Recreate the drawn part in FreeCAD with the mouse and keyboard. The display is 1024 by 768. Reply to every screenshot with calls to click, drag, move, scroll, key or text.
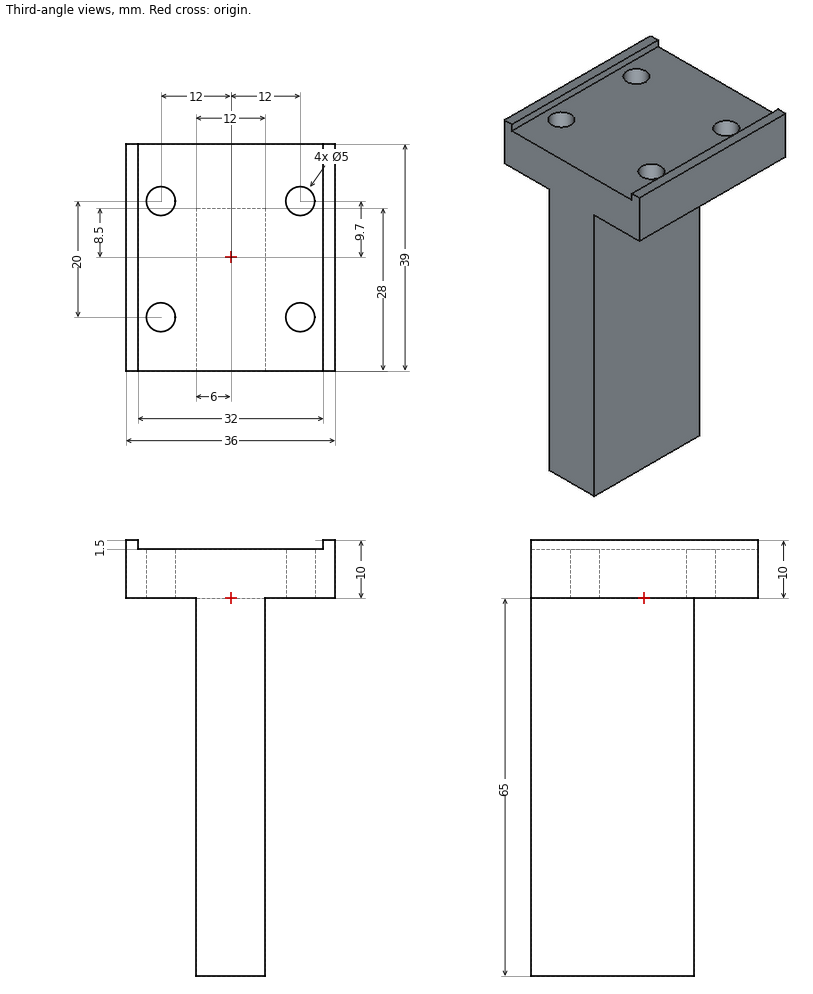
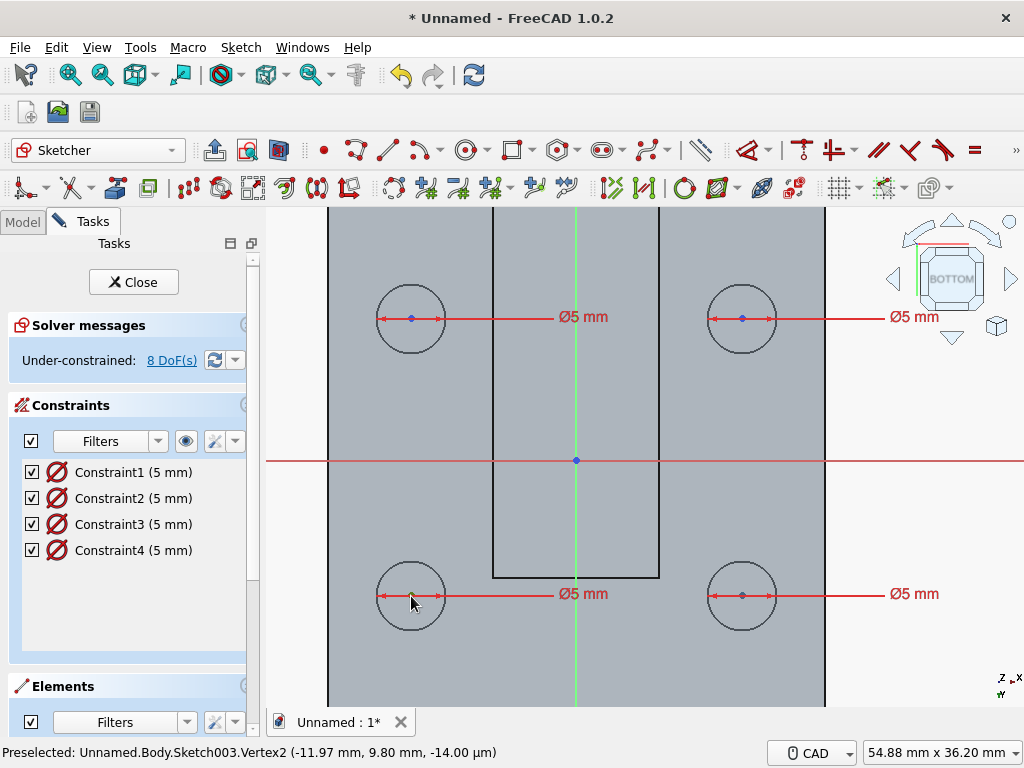
key(h)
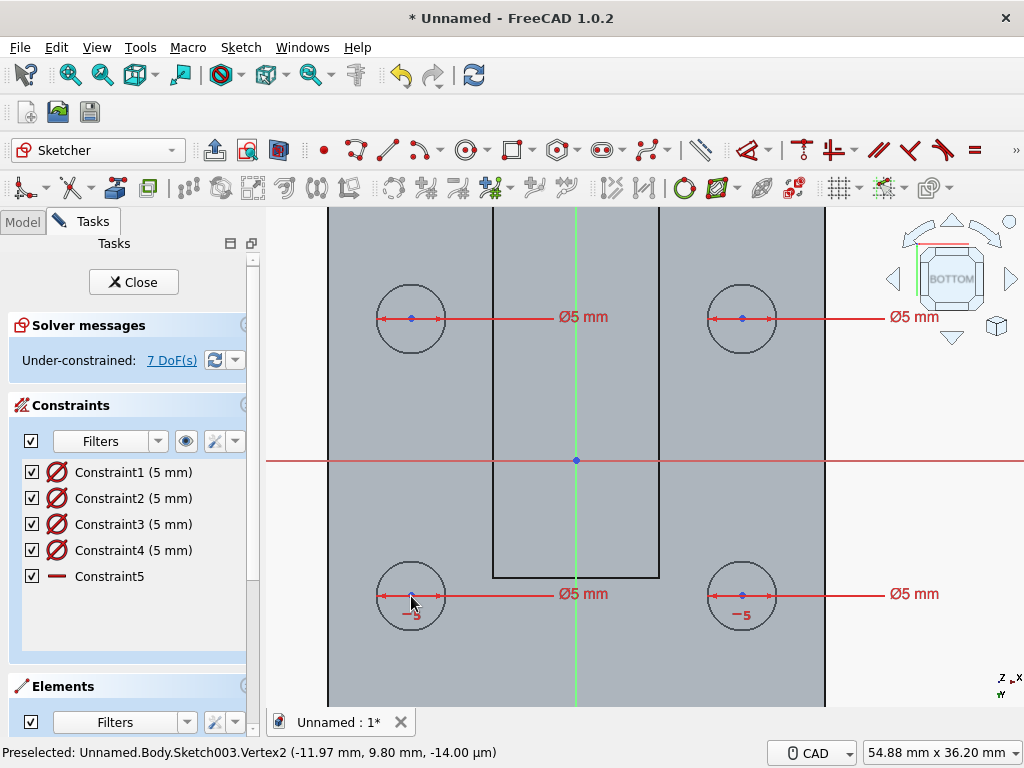
click(411, 596)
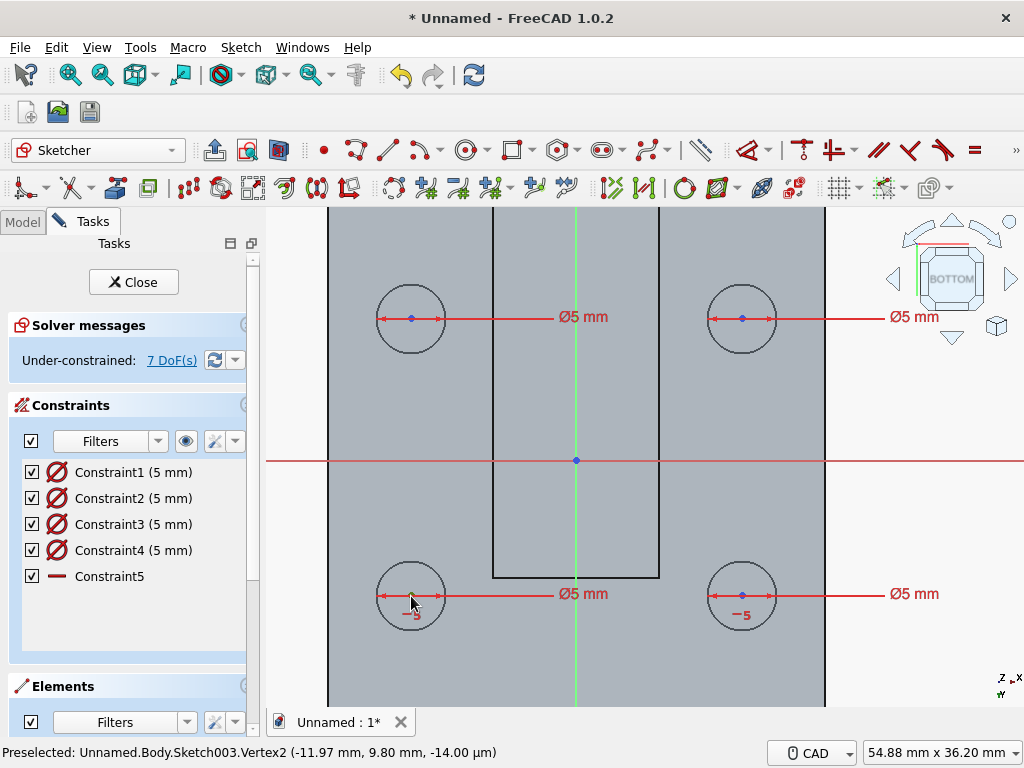
click(411, 319)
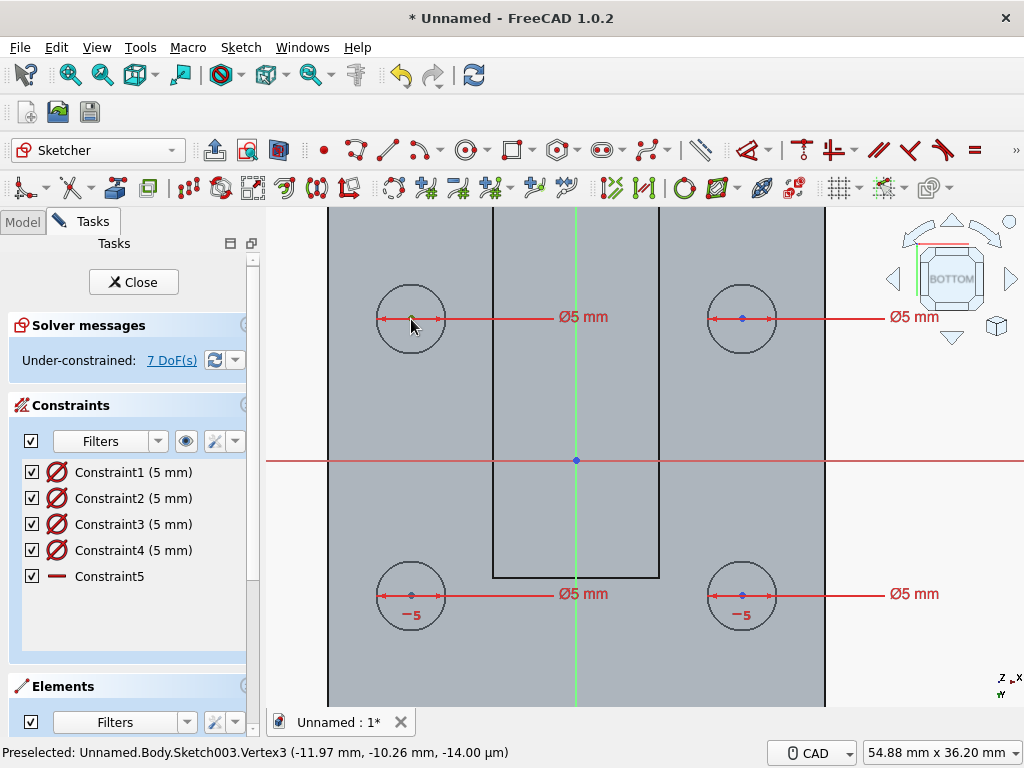
key(v)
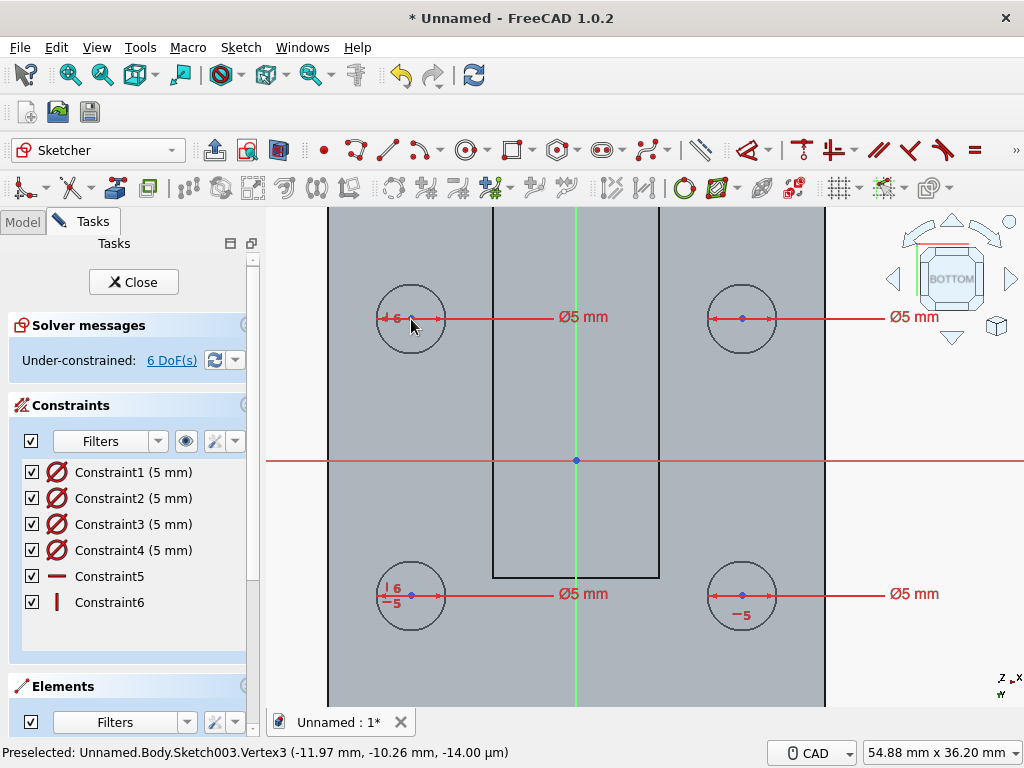
click(742, 596)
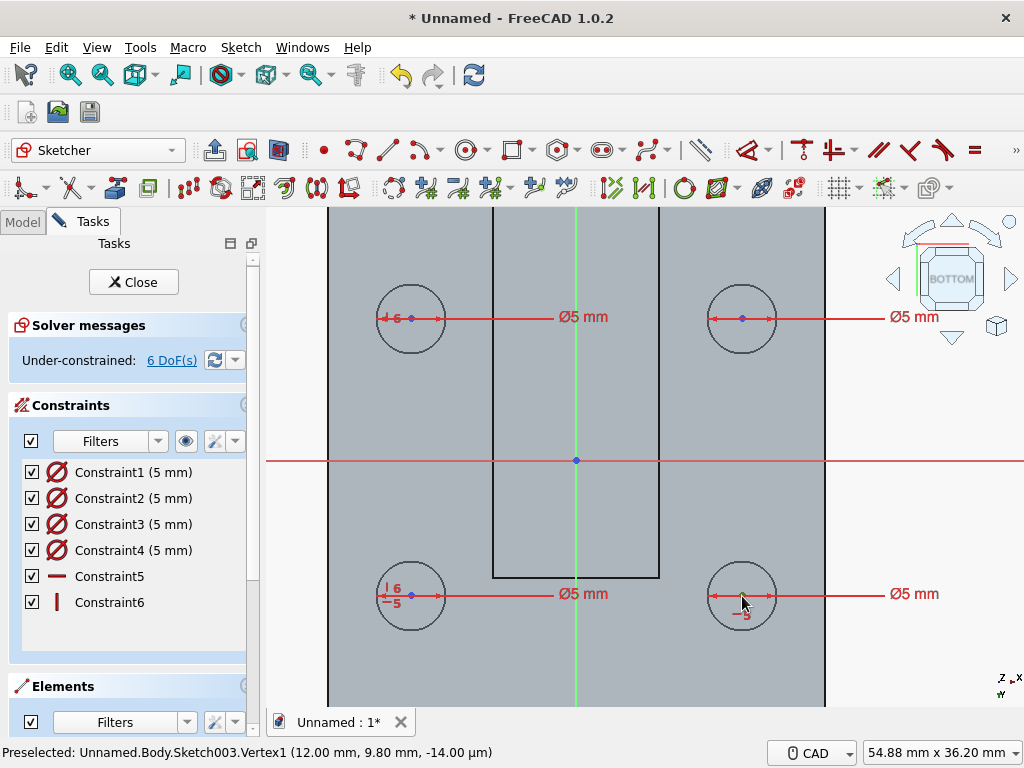
click(742, 319)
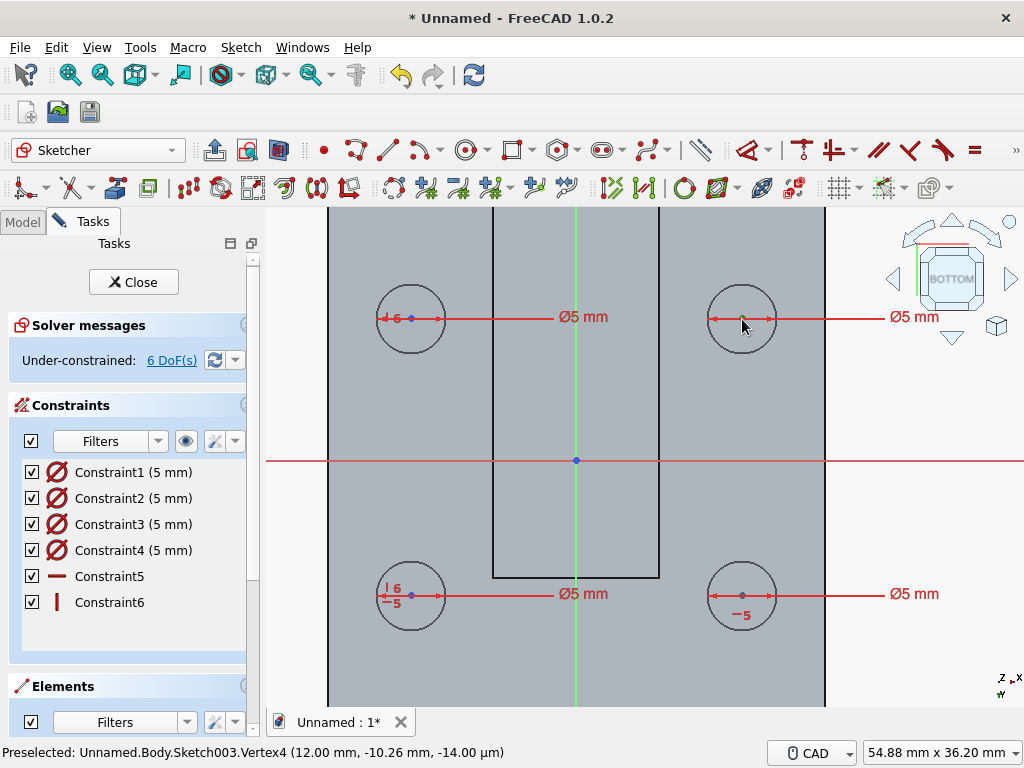
key(v)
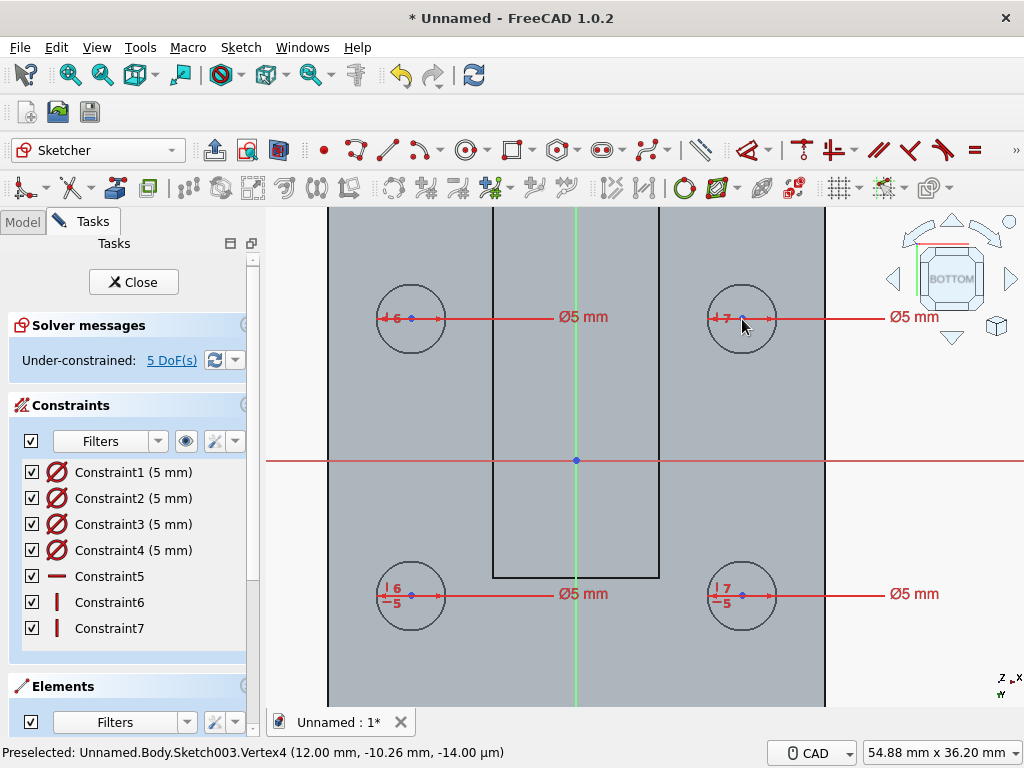
click(411, 319)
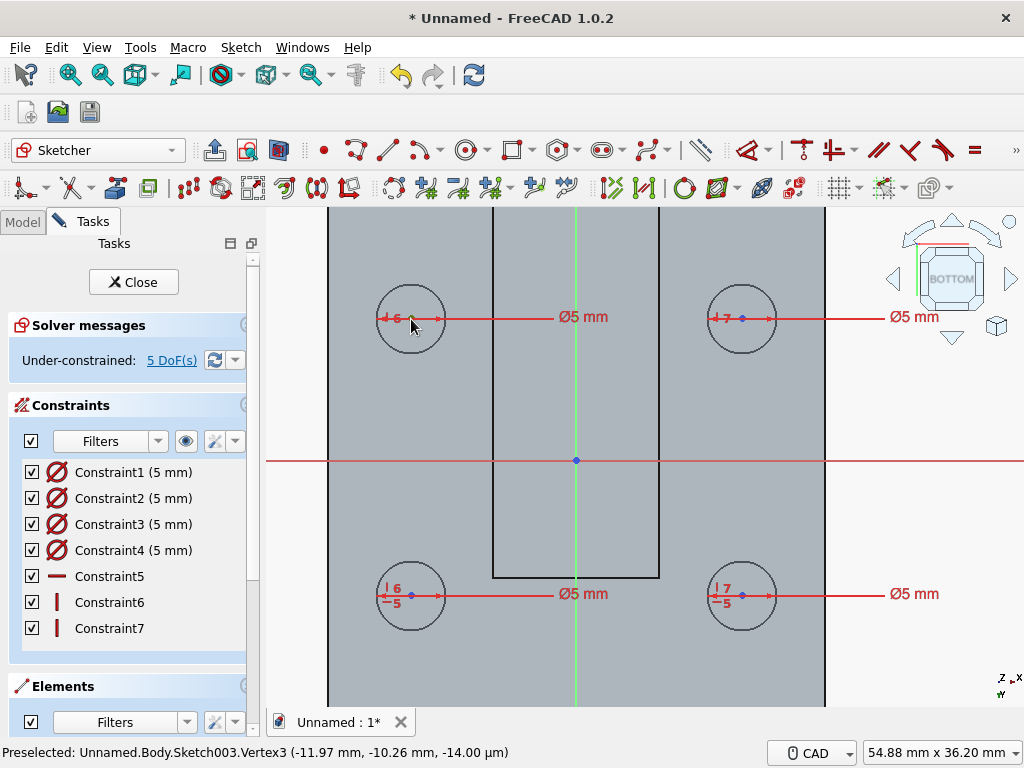
click(742, 319)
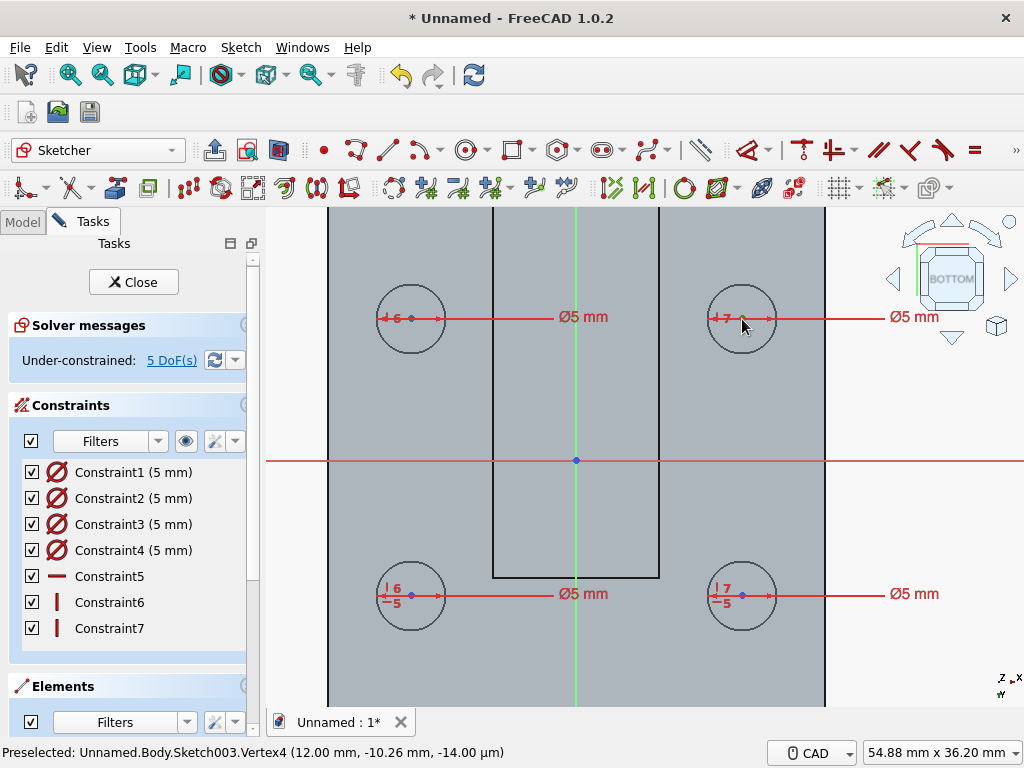
key(h)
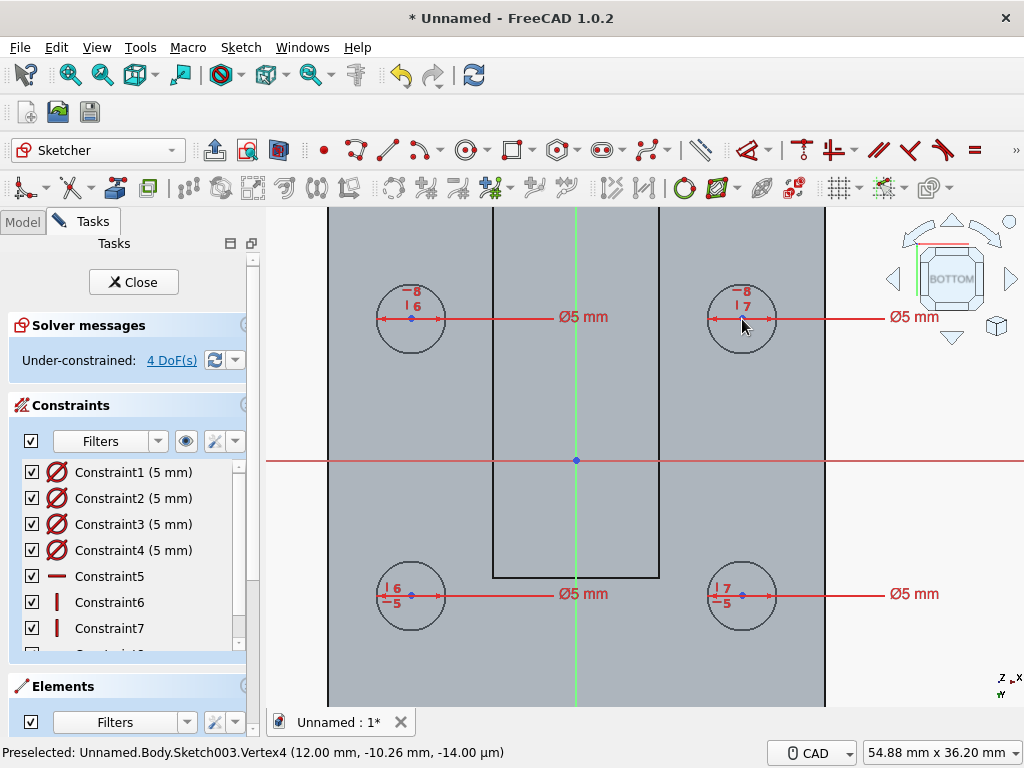
key(d)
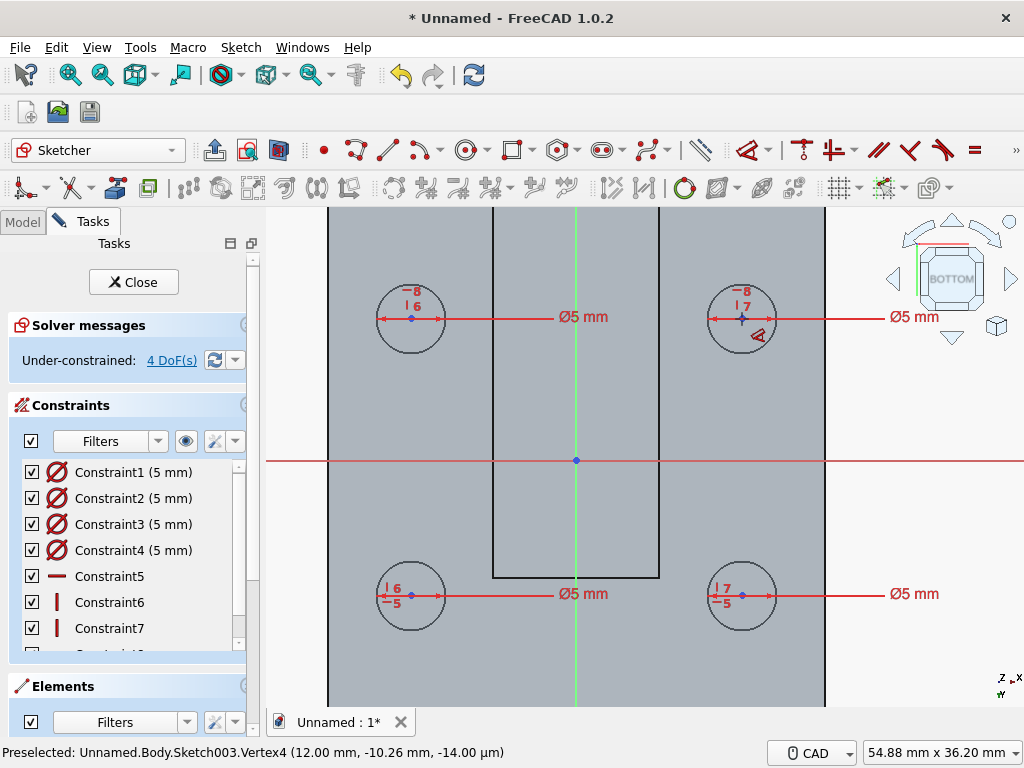
click(742, 596)
click(659, 630)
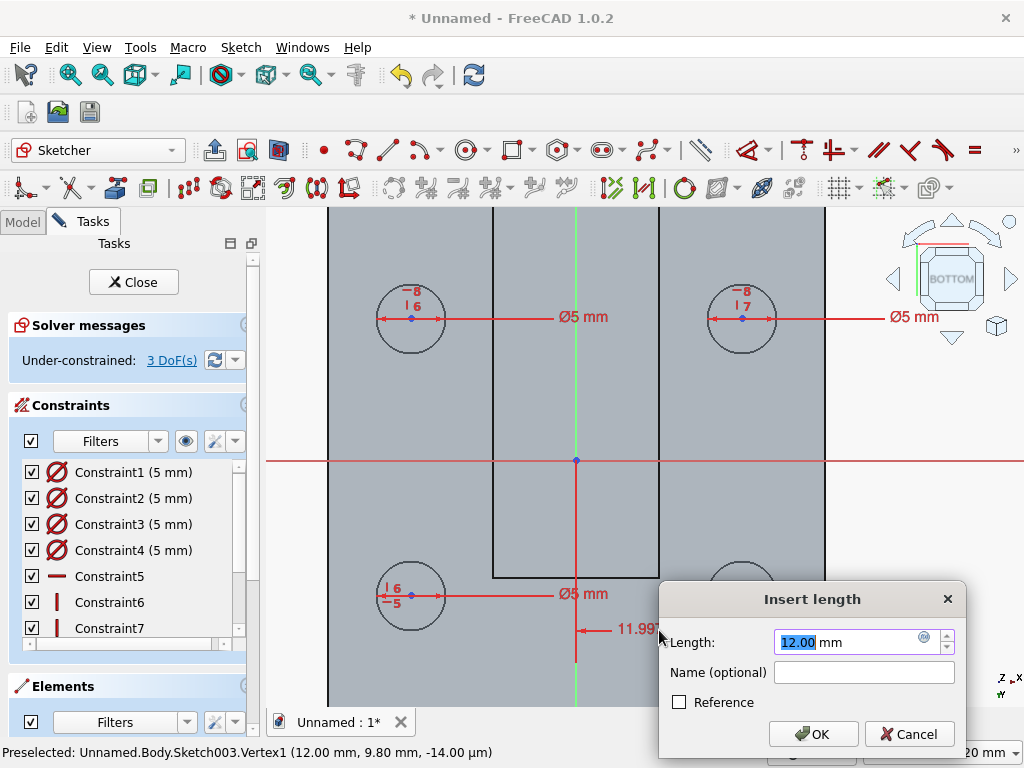
text(12)
key(Return)